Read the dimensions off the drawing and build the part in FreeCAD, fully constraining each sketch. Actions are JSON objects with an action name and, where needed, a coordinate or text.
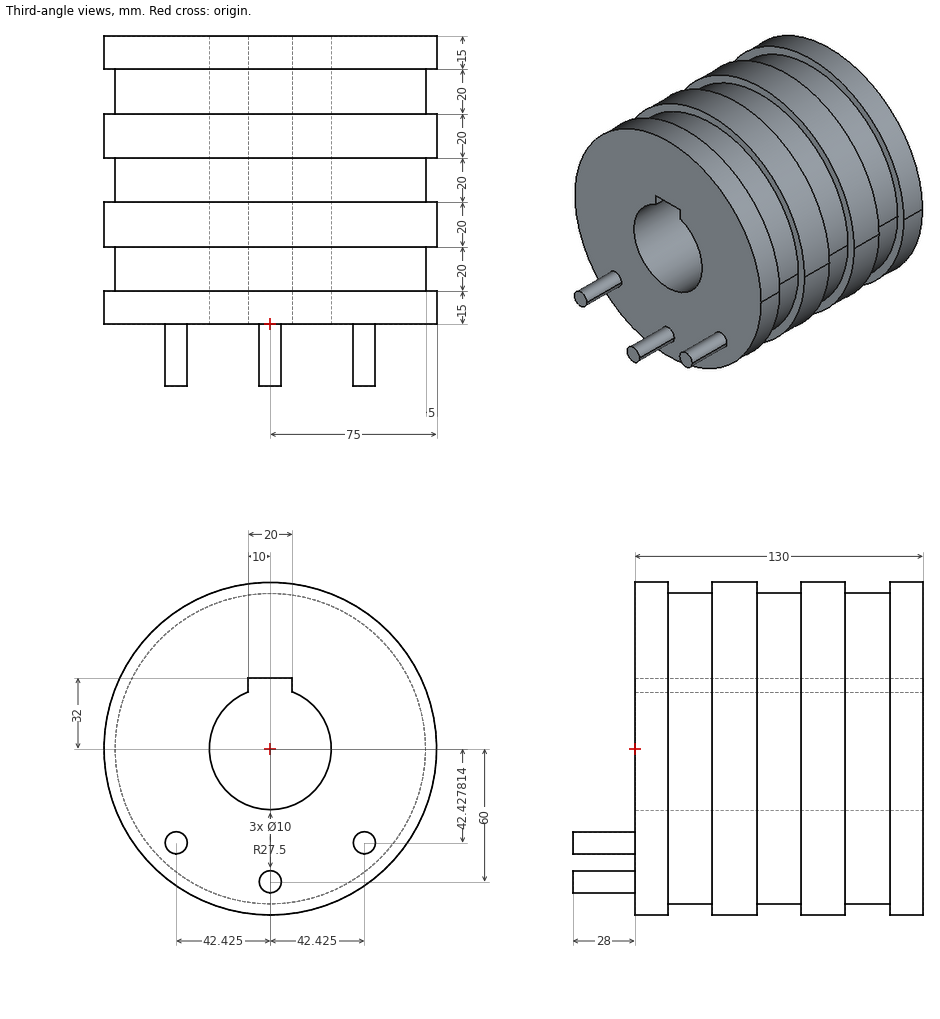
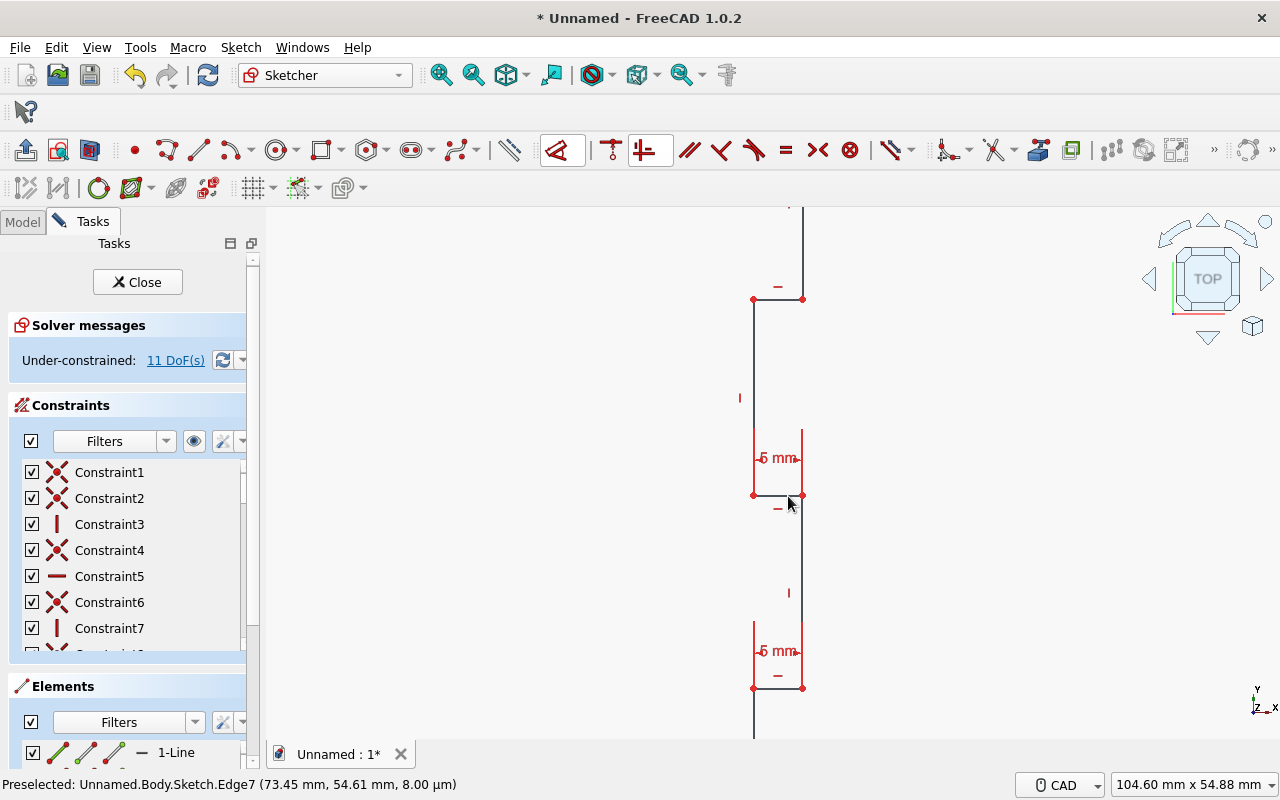
{"action": "left_click", "coordinate": [769, 300]}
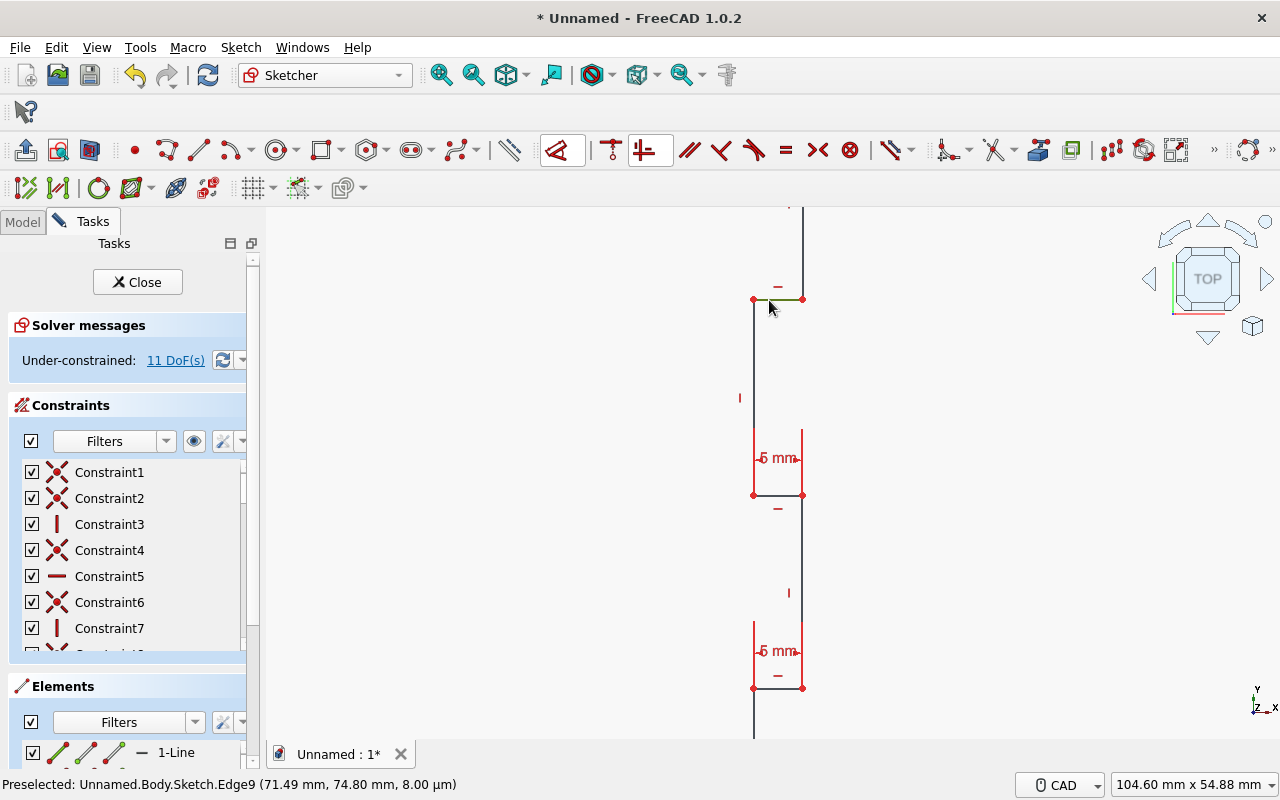
{"action": "key", "text": "l"}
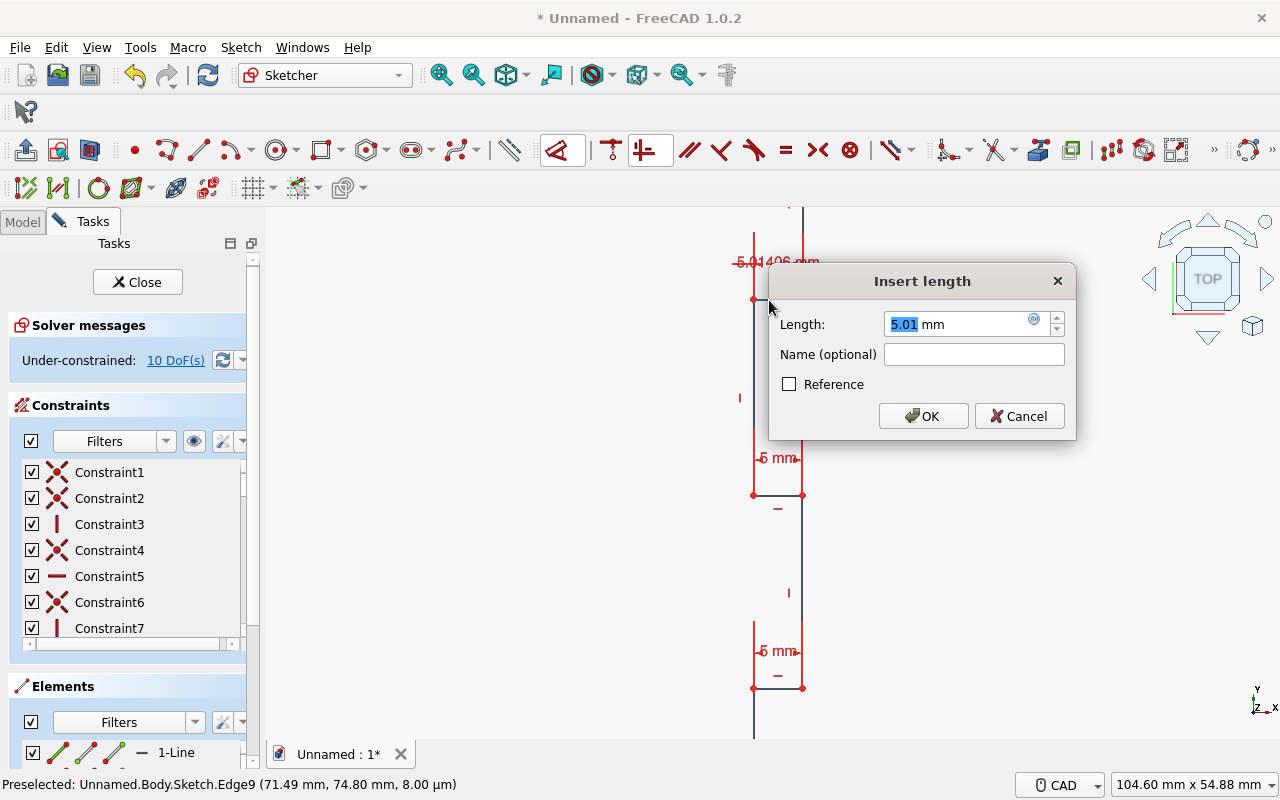
{"action": "type", "text": "5"}
{"action": "key", "text": "Return"}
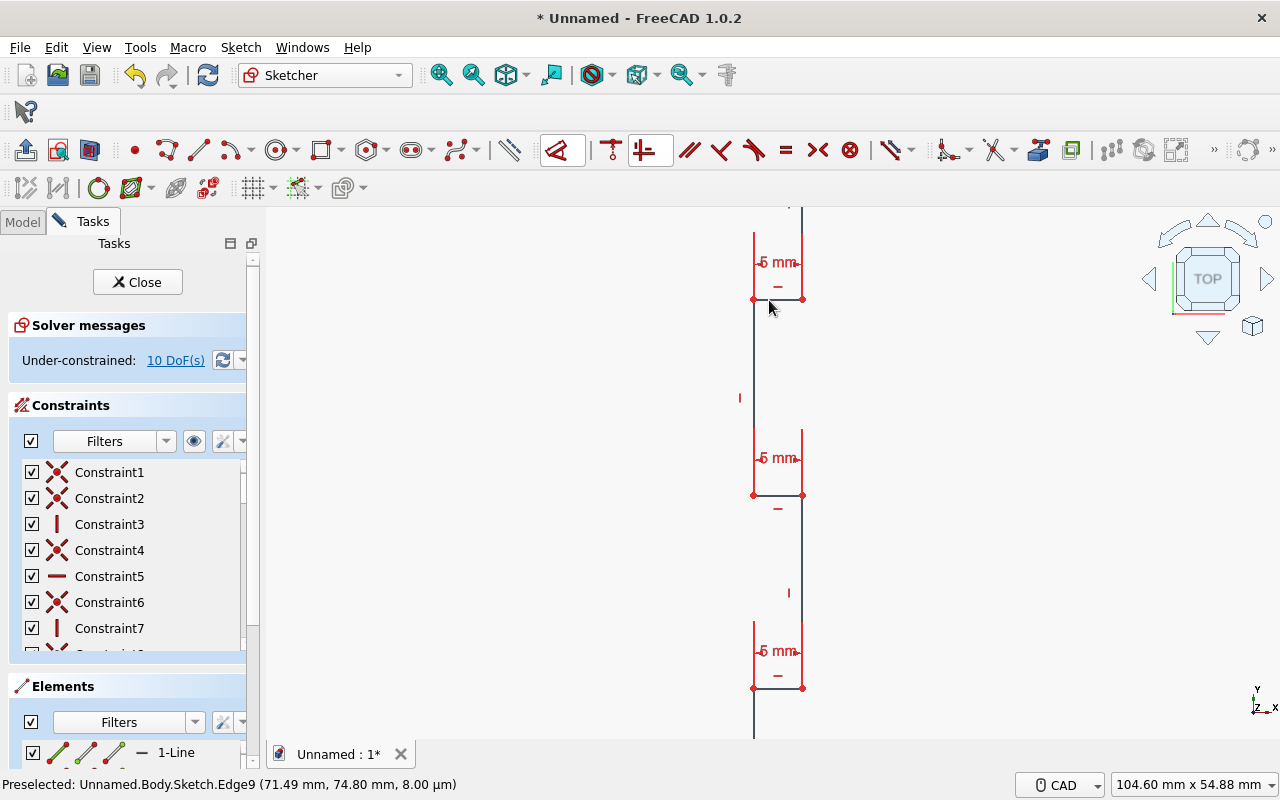
{"action": "scroll", "coordinate": [791, 499], "scroll_direction": "down", "scroll_amount": 7}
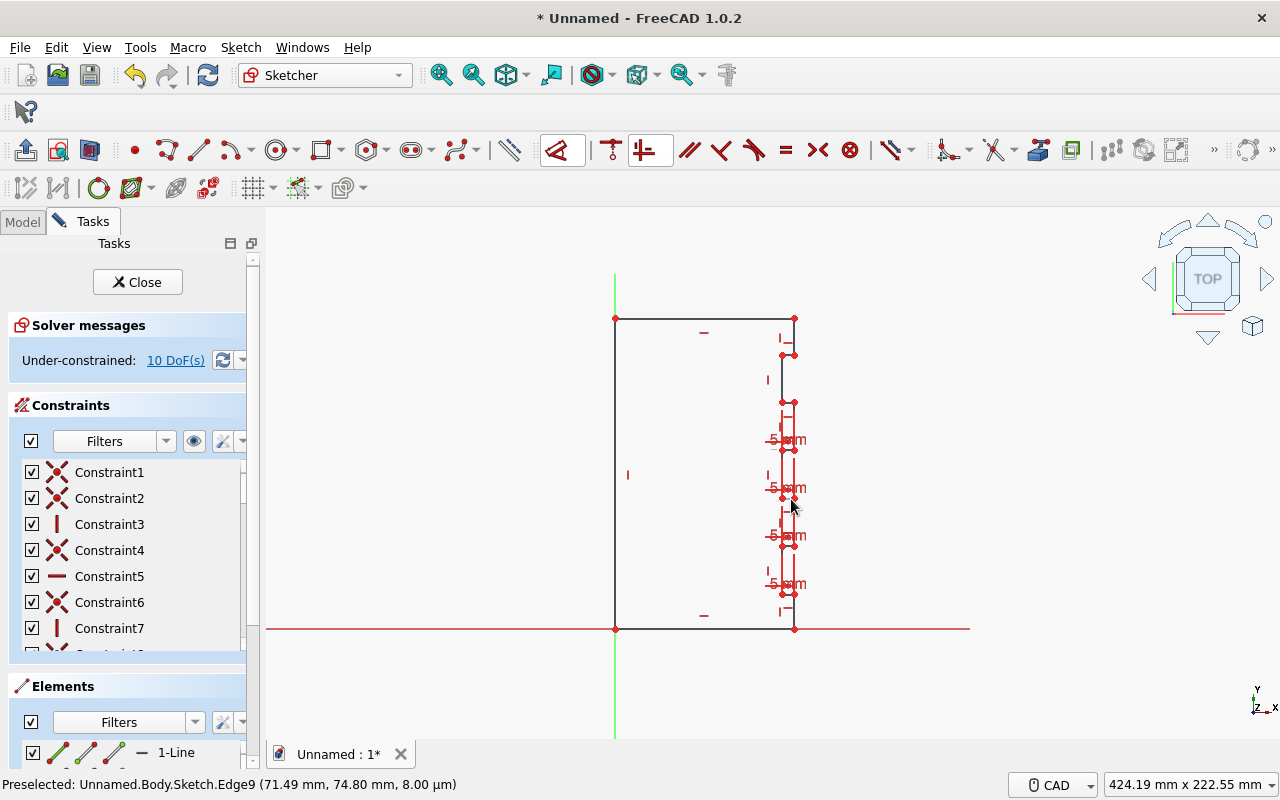
{"action": "scroll", "coordinate": [791, 403], "scroll_direction": "up", "scroll_amount": 7}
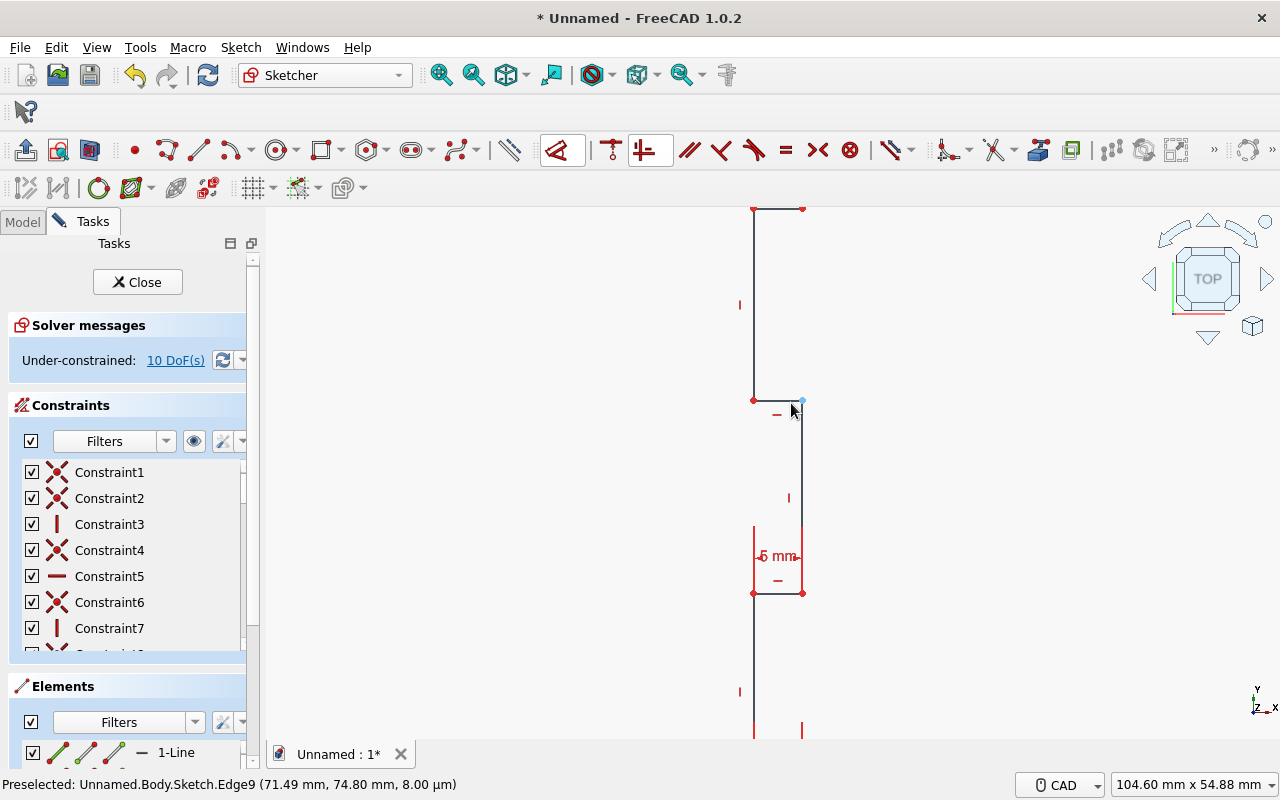
{"action": "left_click", "coordinate": [788, 401]}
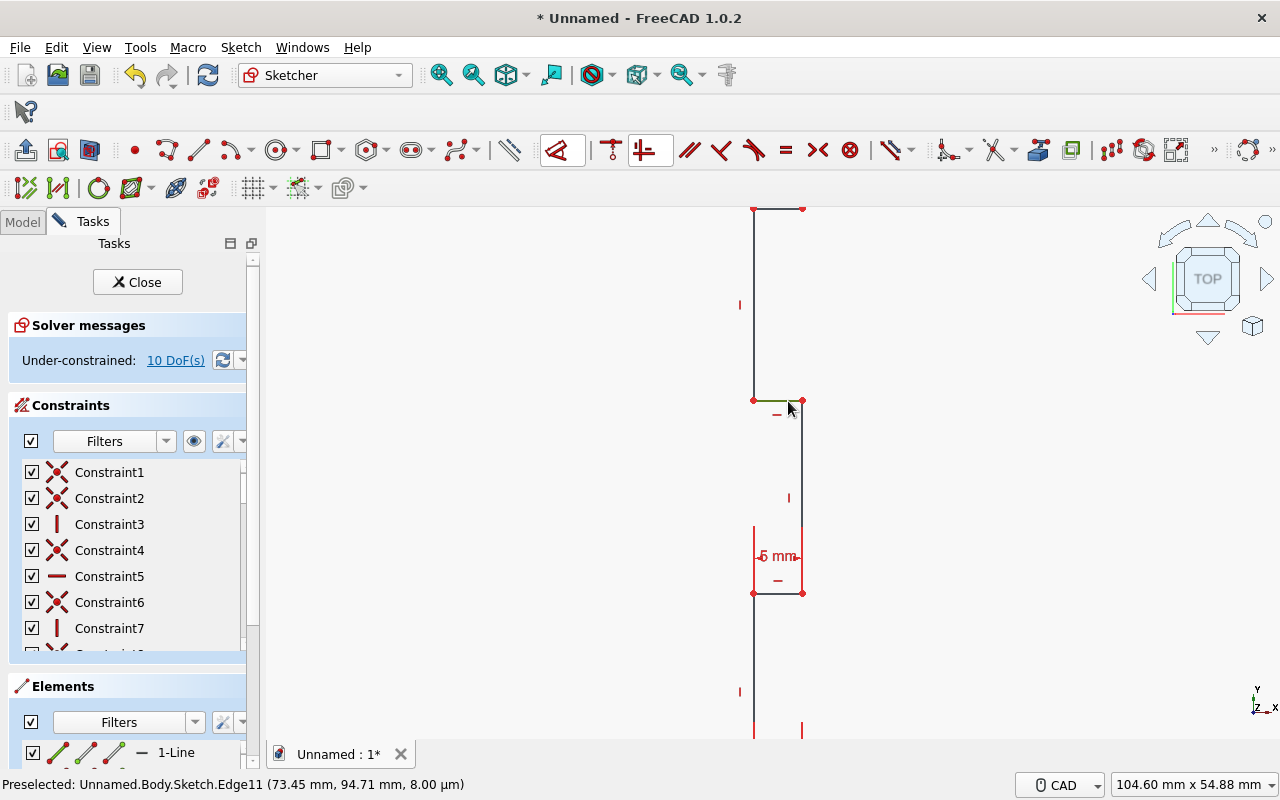
{"action": "key", "text": "l"}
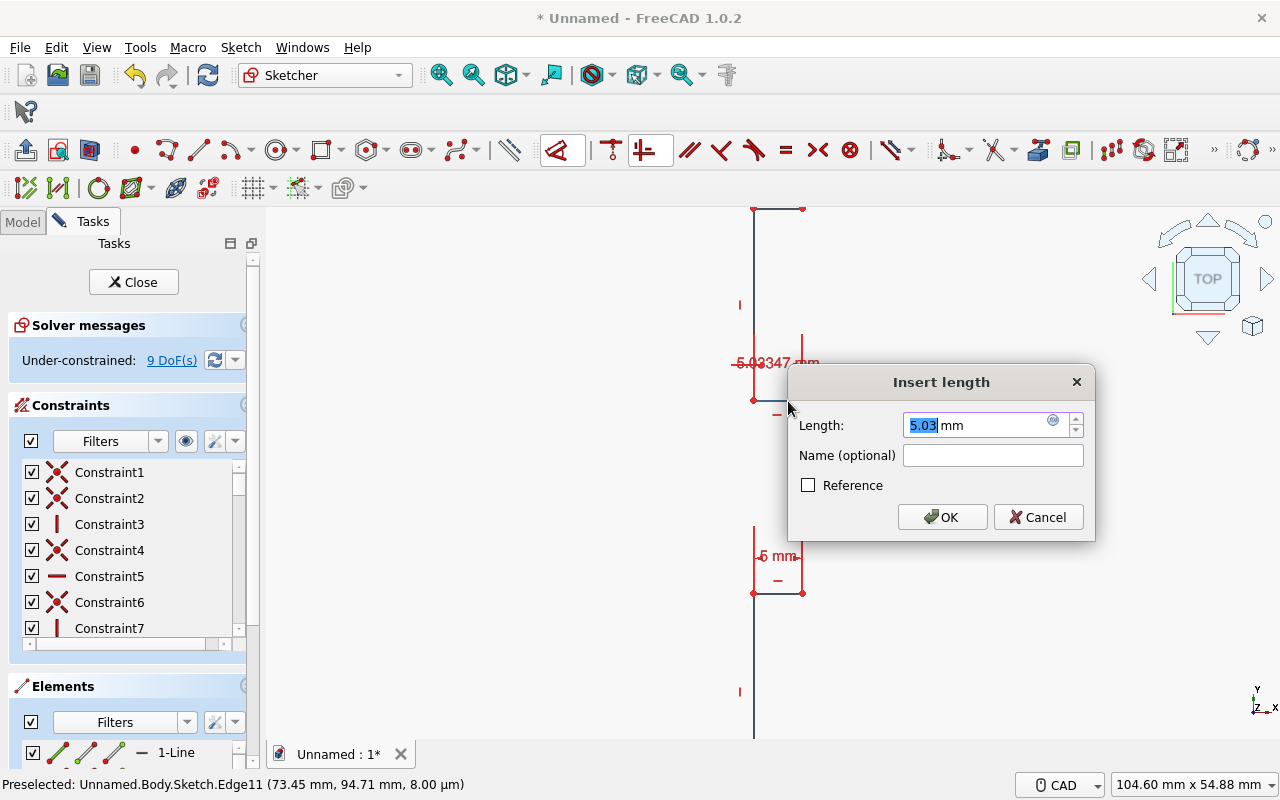
{"action": "type", "text": "5"}
{"action": "key", "text": "Return"}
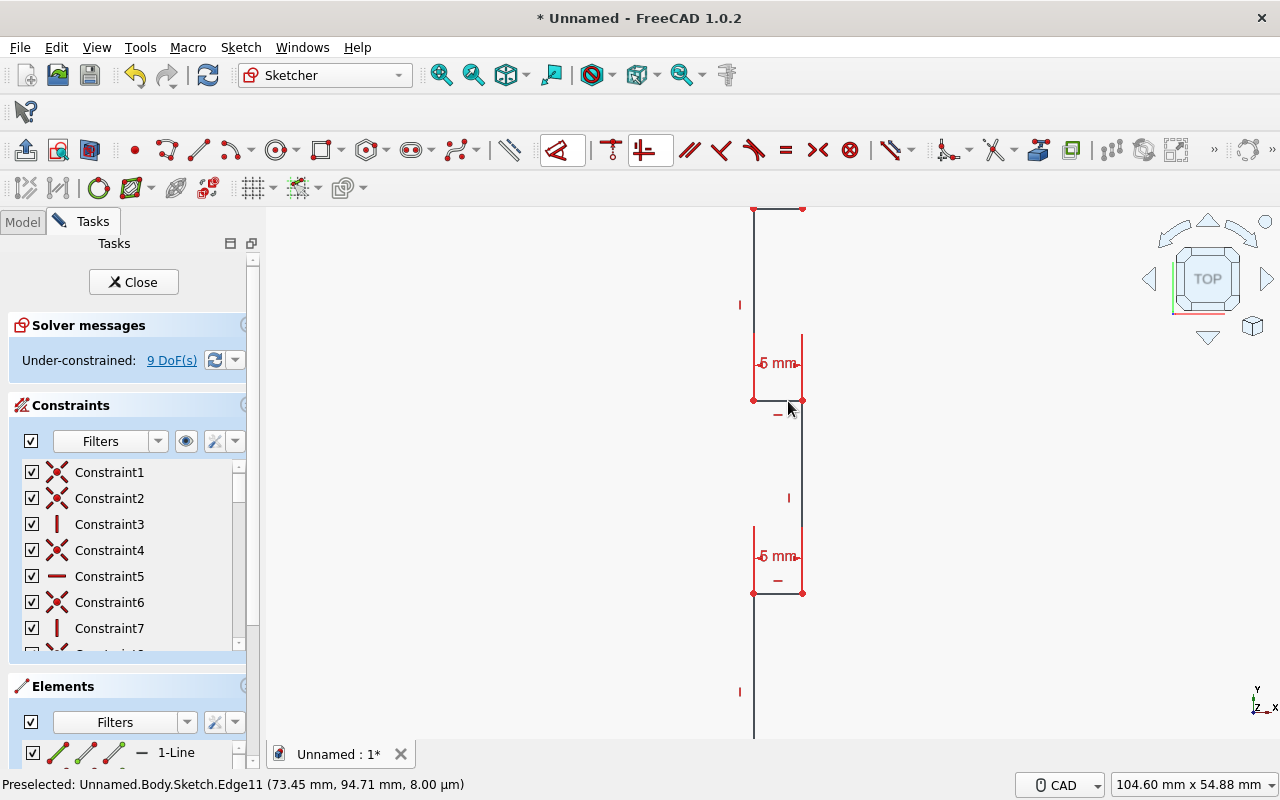
{"action": "scroll", "coordinate": [791, 402], "scroll_direction": "down", "scroll_amount": 7}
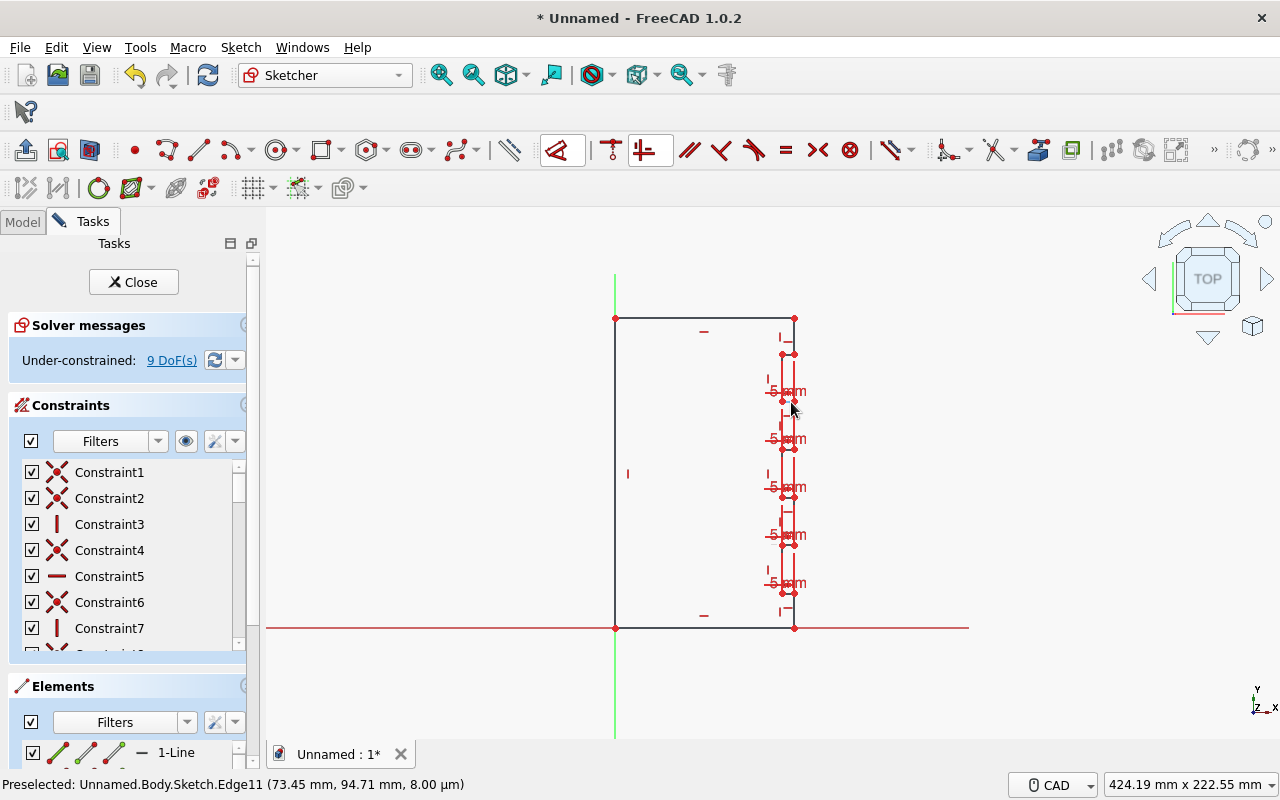
{"action": "scroll", "coordinate": [786, 355], "scroll_direction": "up", "scroll_amount": 7}